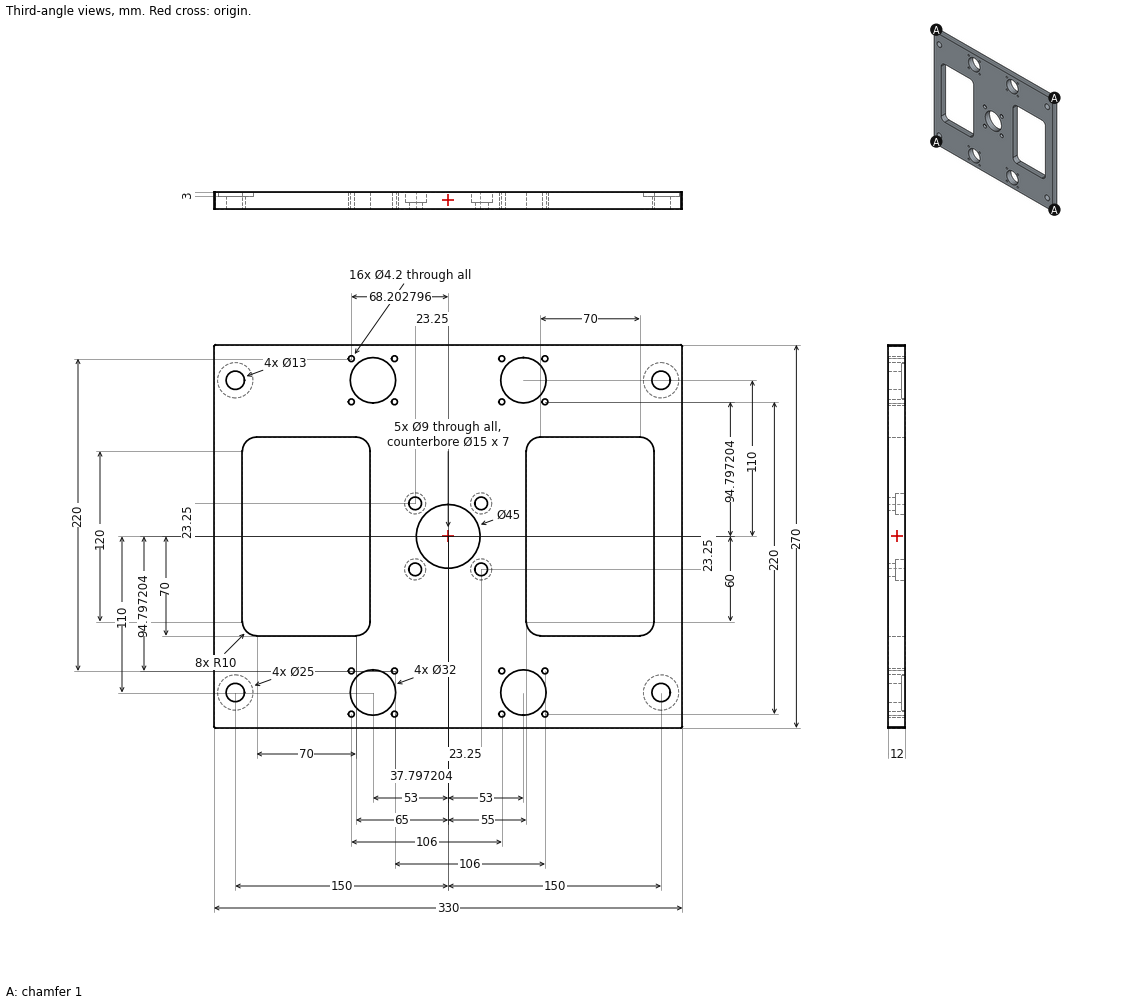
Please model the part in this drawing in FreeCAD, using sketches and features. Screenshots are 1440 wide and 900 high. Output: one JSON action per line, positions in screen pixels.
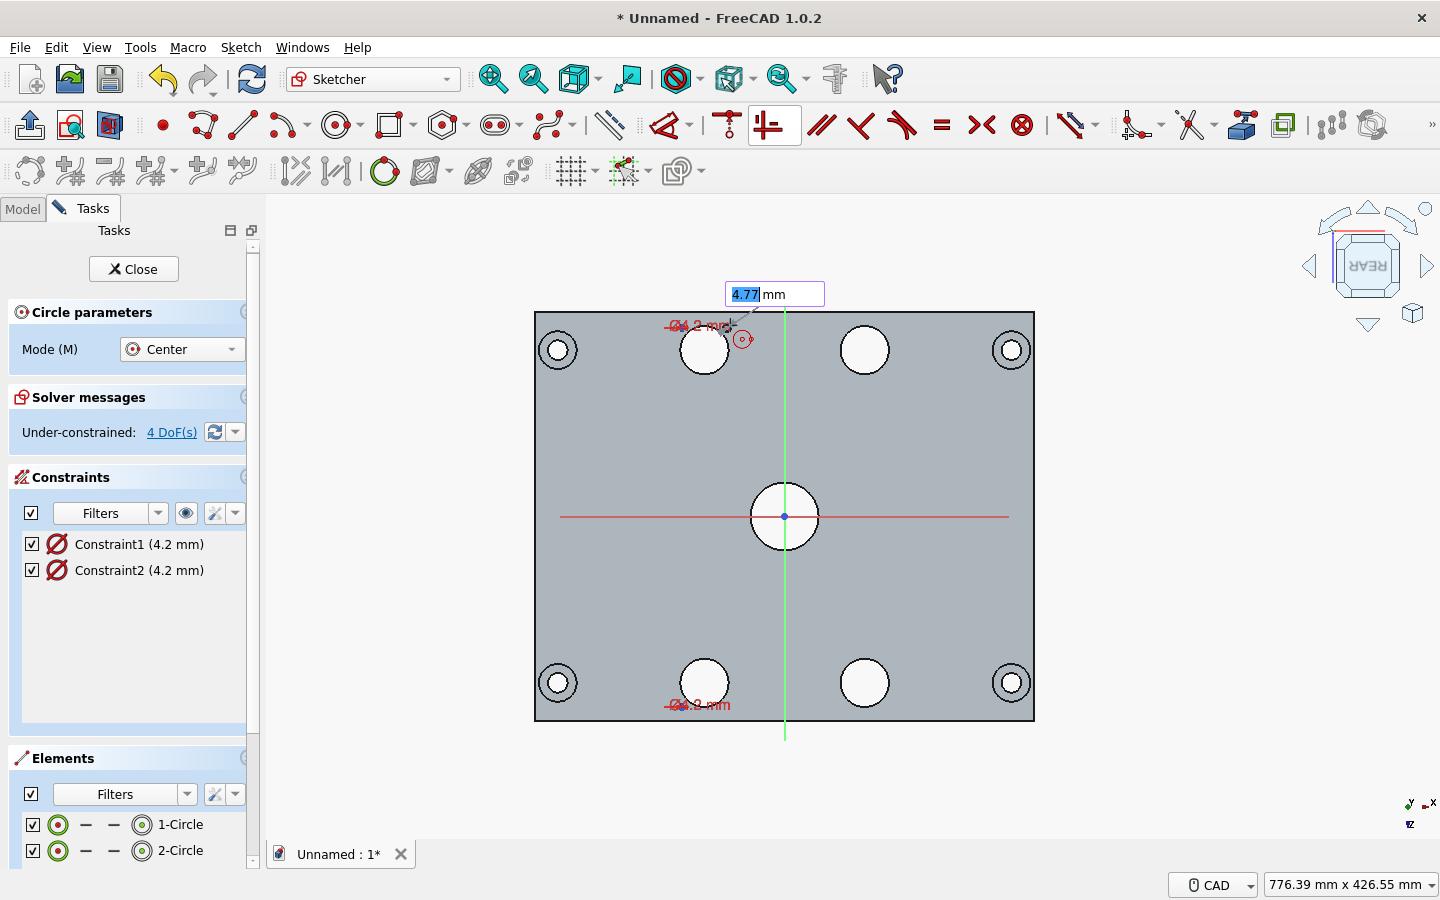
{"action": "type", "text": "4.2"}
{"action": "key", "text": "Return"}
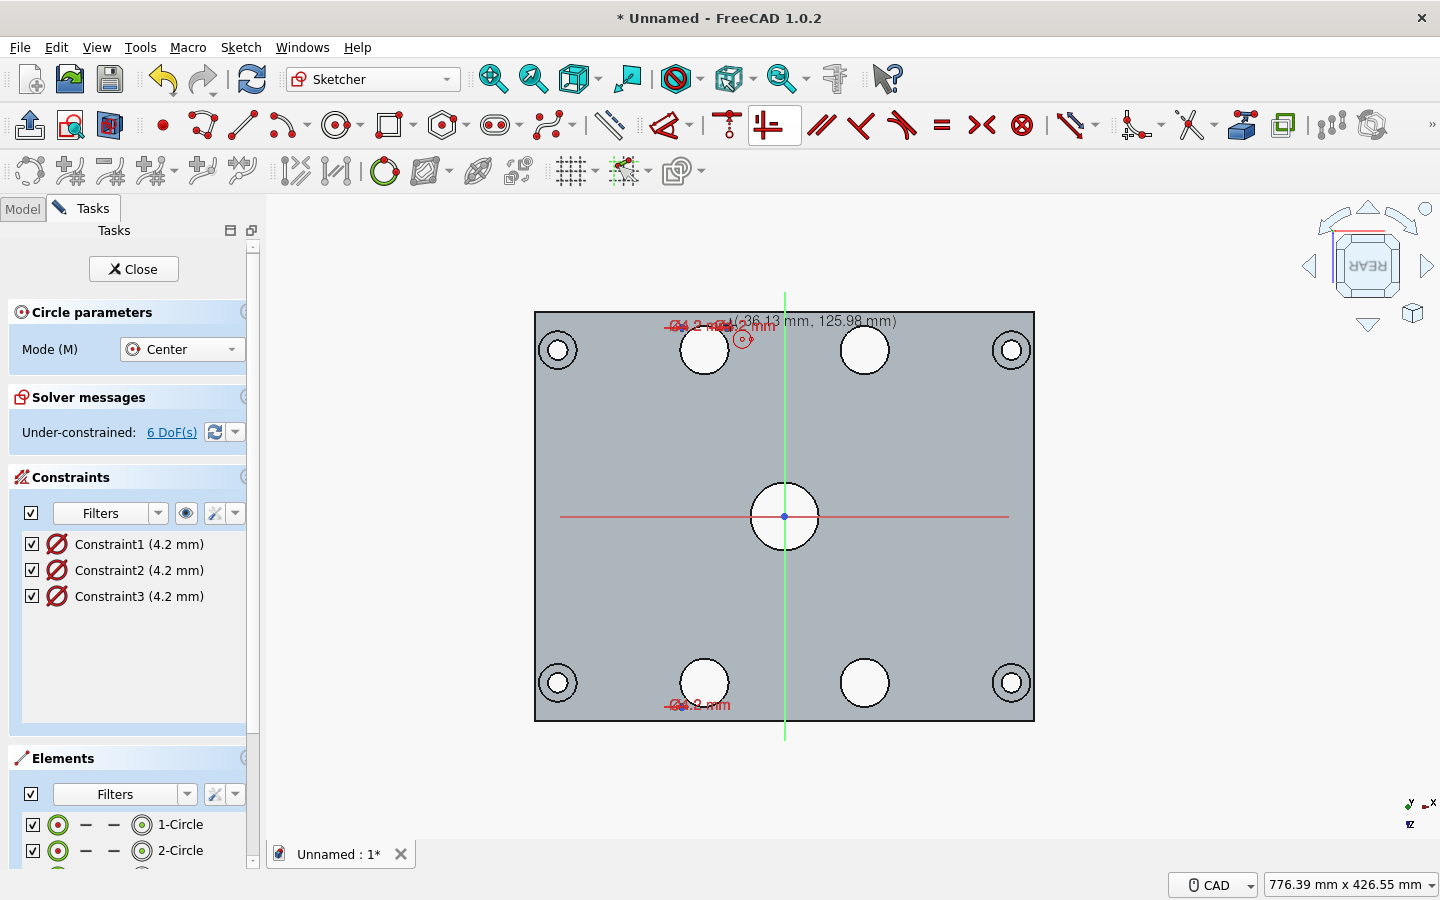
{"action": "scroll", "coordinate": [727, 373], "scroll_direction": "up", "scroll_amount": 10}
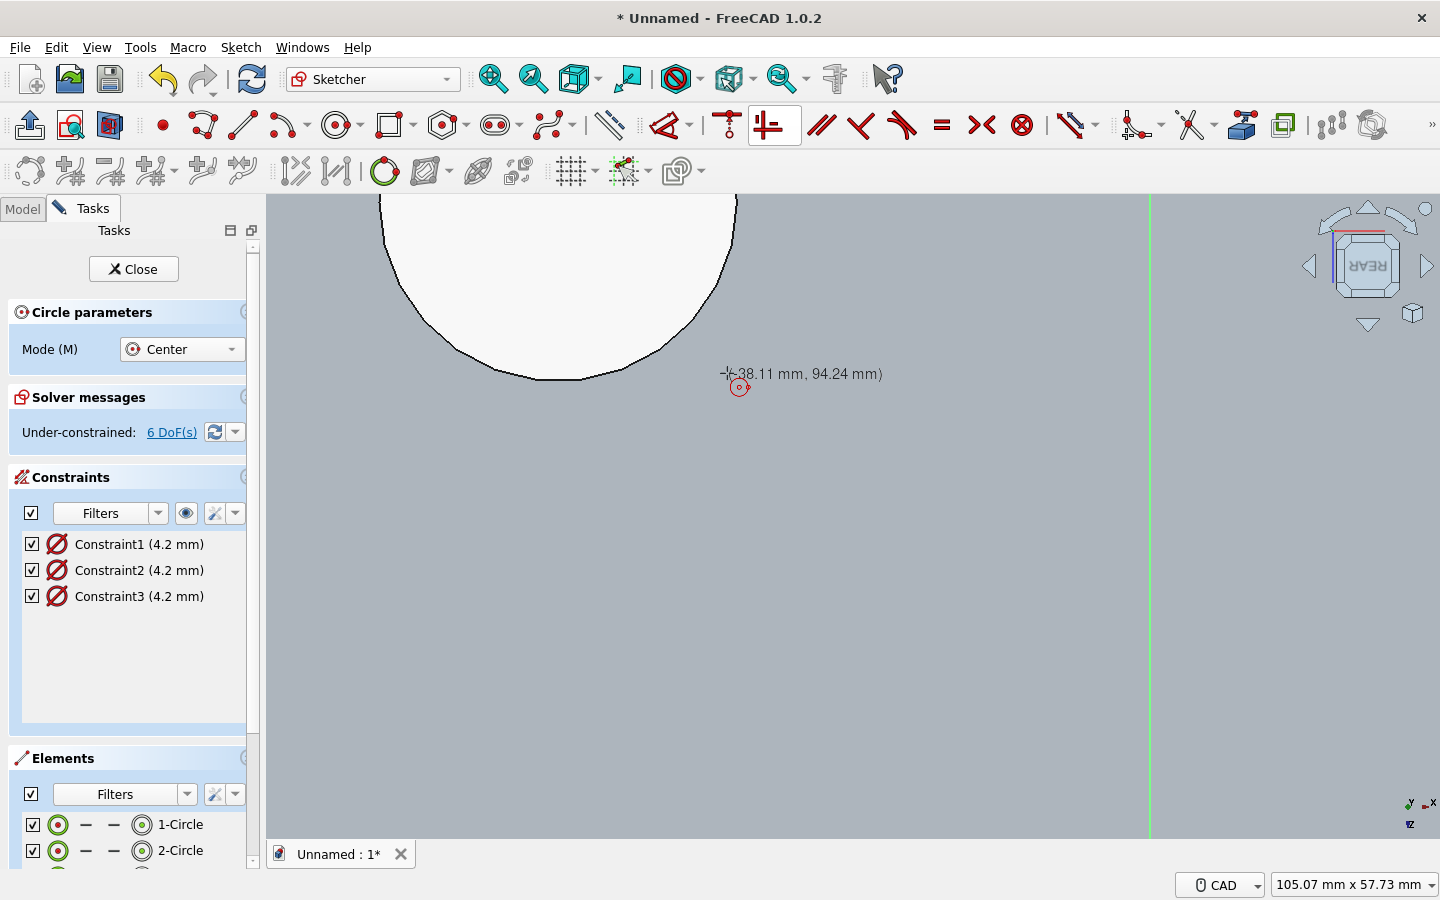
{"action": "scroll", "coordinate": [727, 373], "scroll_direction": "down", "scroll_amount": 10}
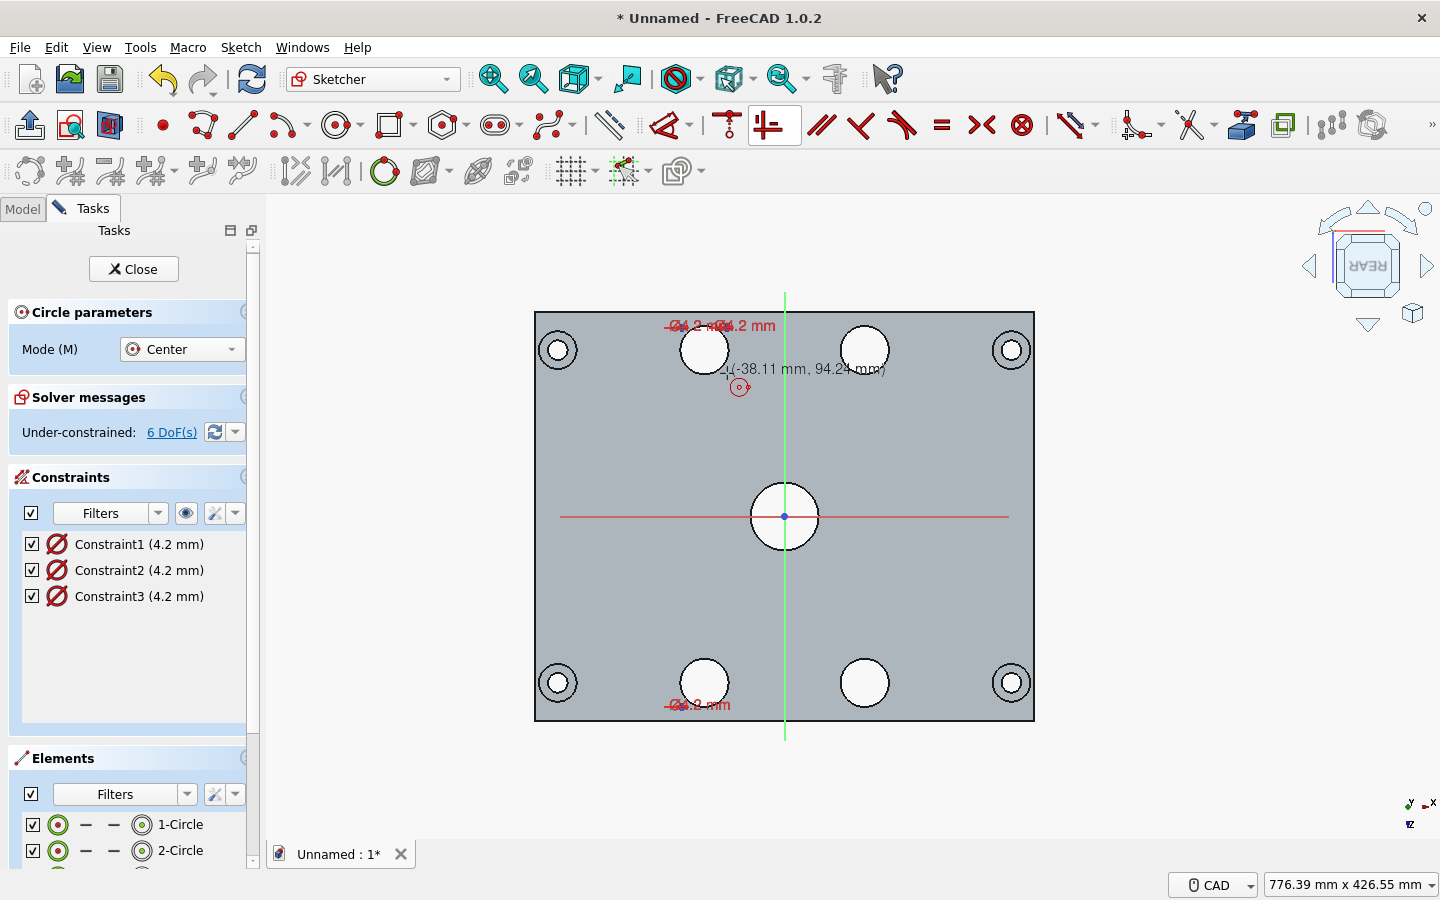
{"action": "left_click", "coordinate": [727, 373]}
{"action": "mouse_move", "coordinate": [730, 371]}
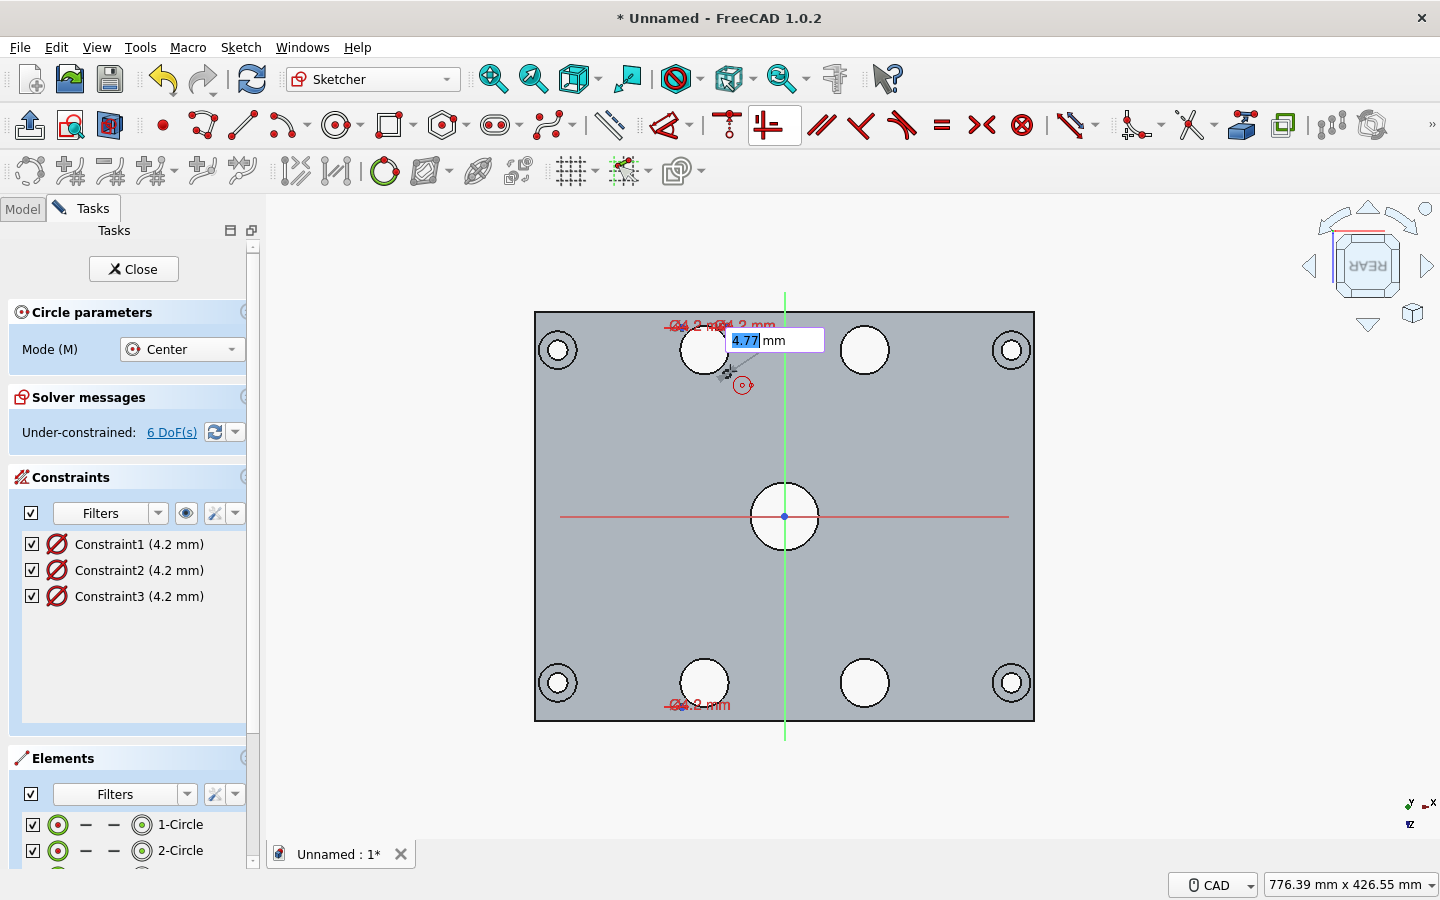
{"action": "type", "text": "4.2"}
{"action": "key", "text": "Return"}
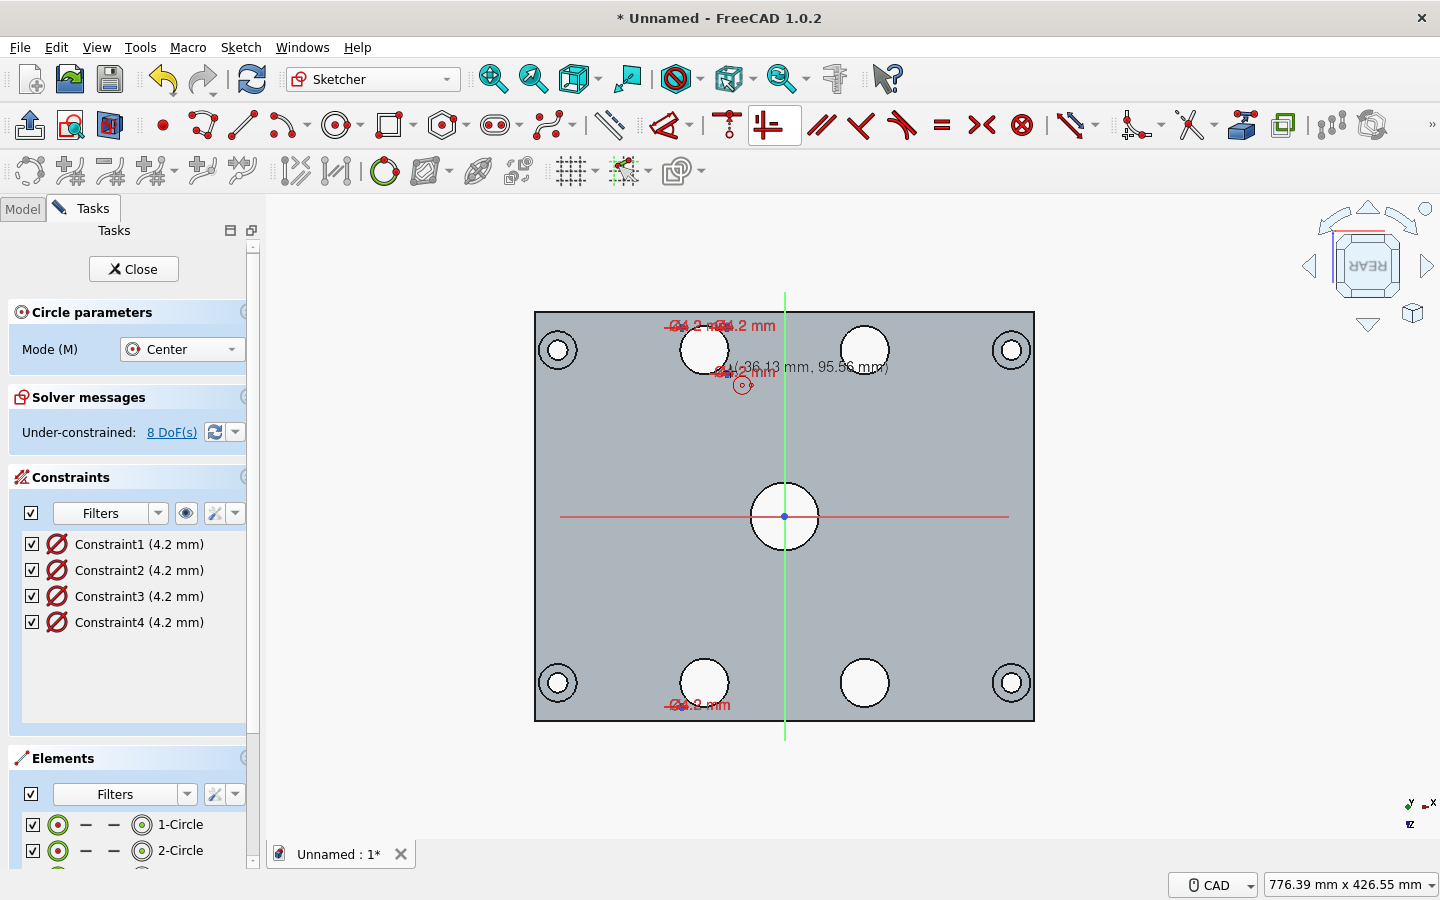
{"action": "scroll", "coordinate": [682, 373], "scroll_direction": "up", "scroll_amount": 10}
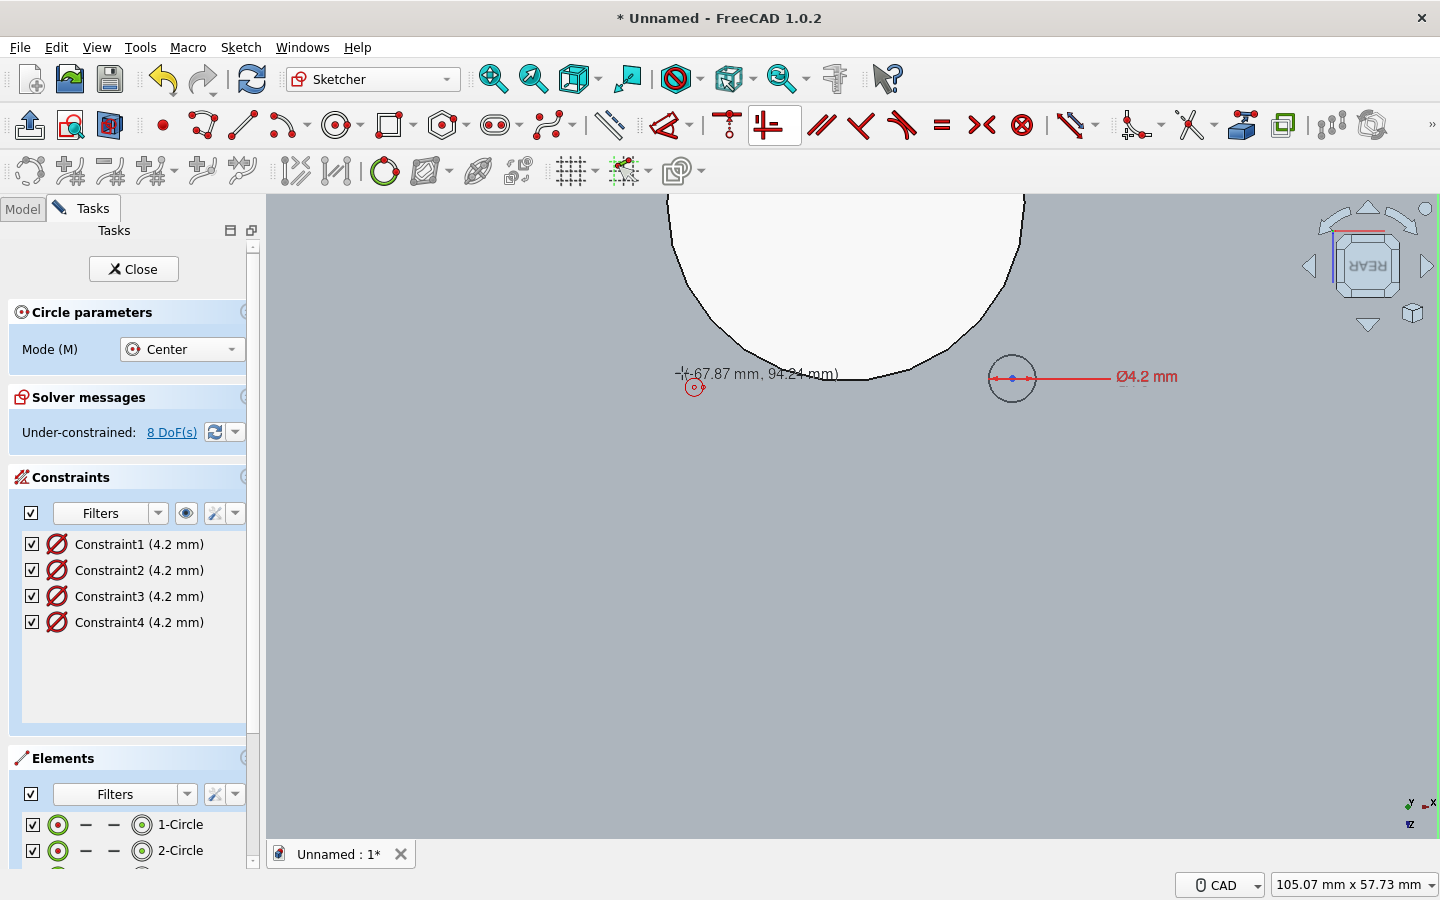
{"action": "scroll", "coordinate": [682, 373], "scroll_direction": "down", "scroll_amount": 10}